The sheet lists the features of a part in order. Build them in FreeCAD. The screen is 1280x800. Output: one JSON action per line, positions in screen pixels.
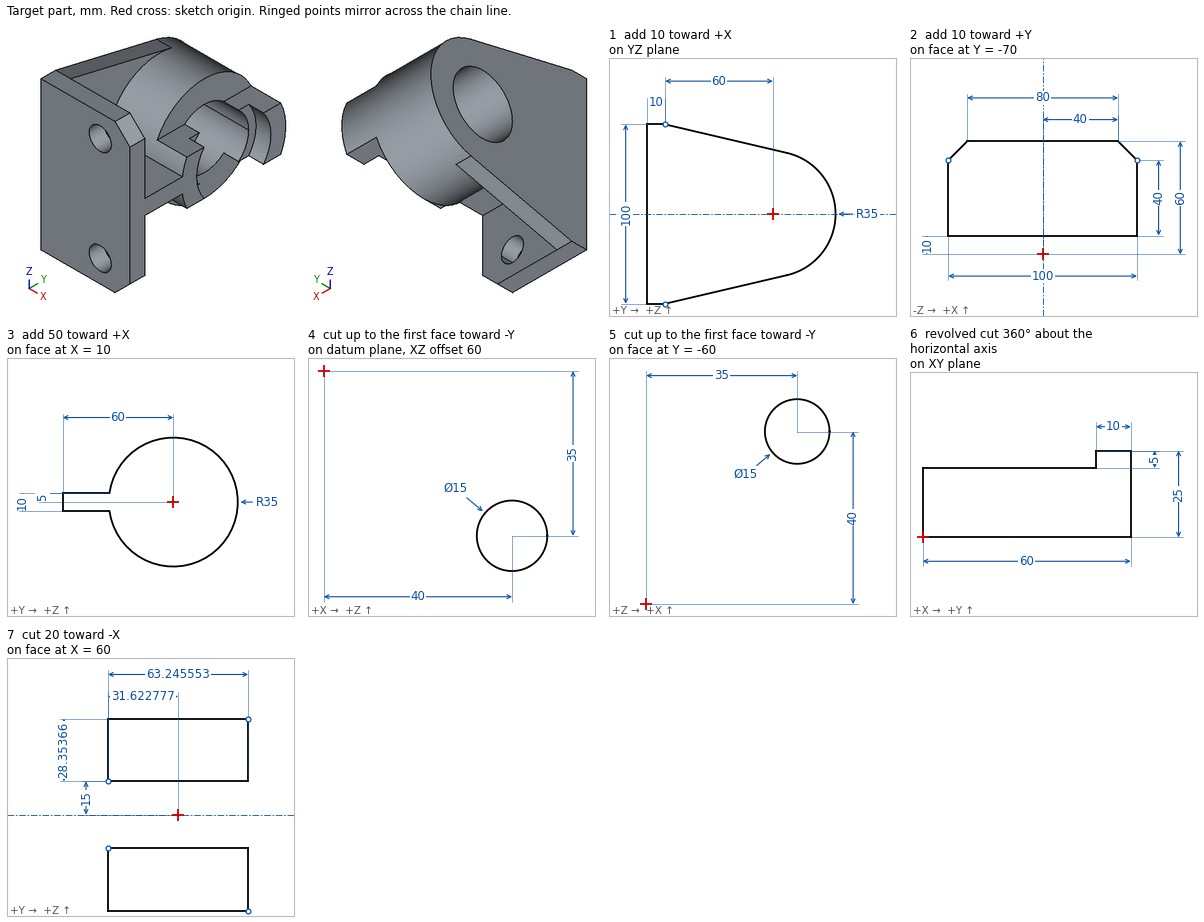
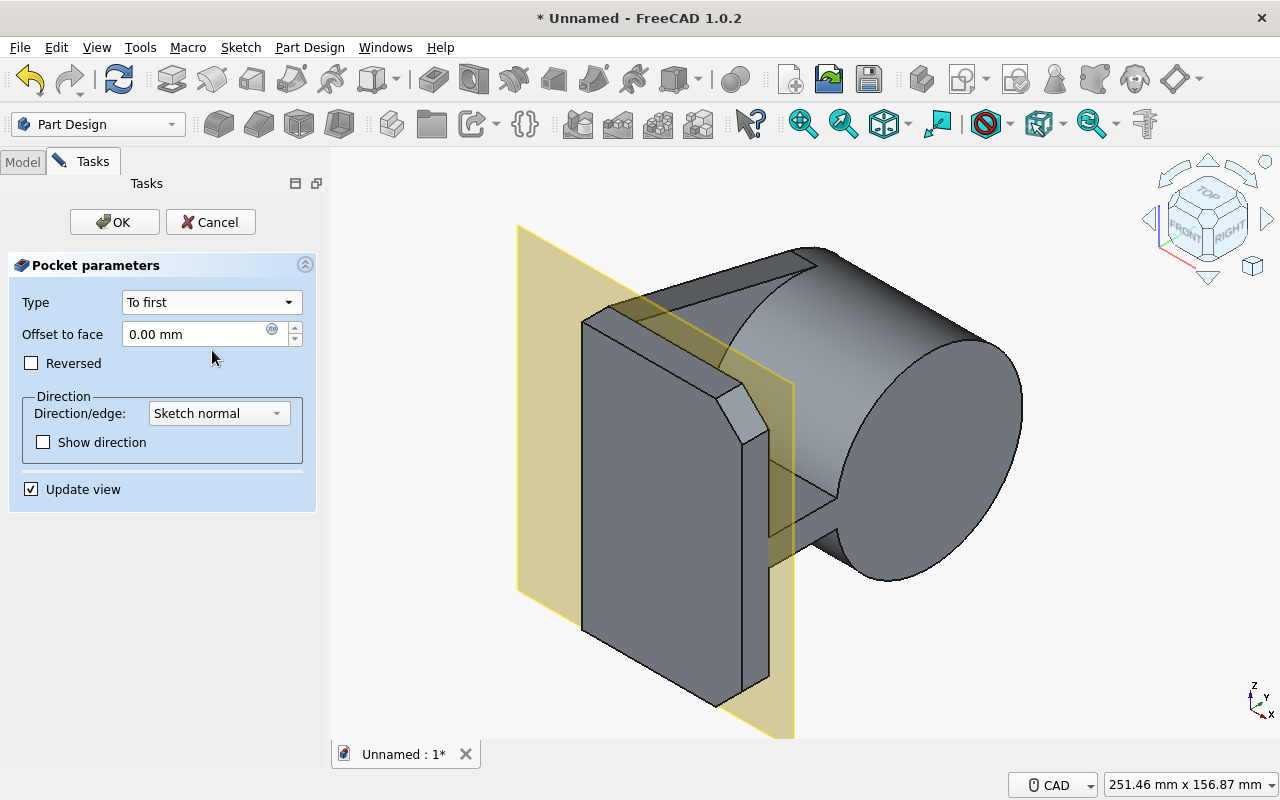
{"action": "left_click", "coordinate": [30, 363]}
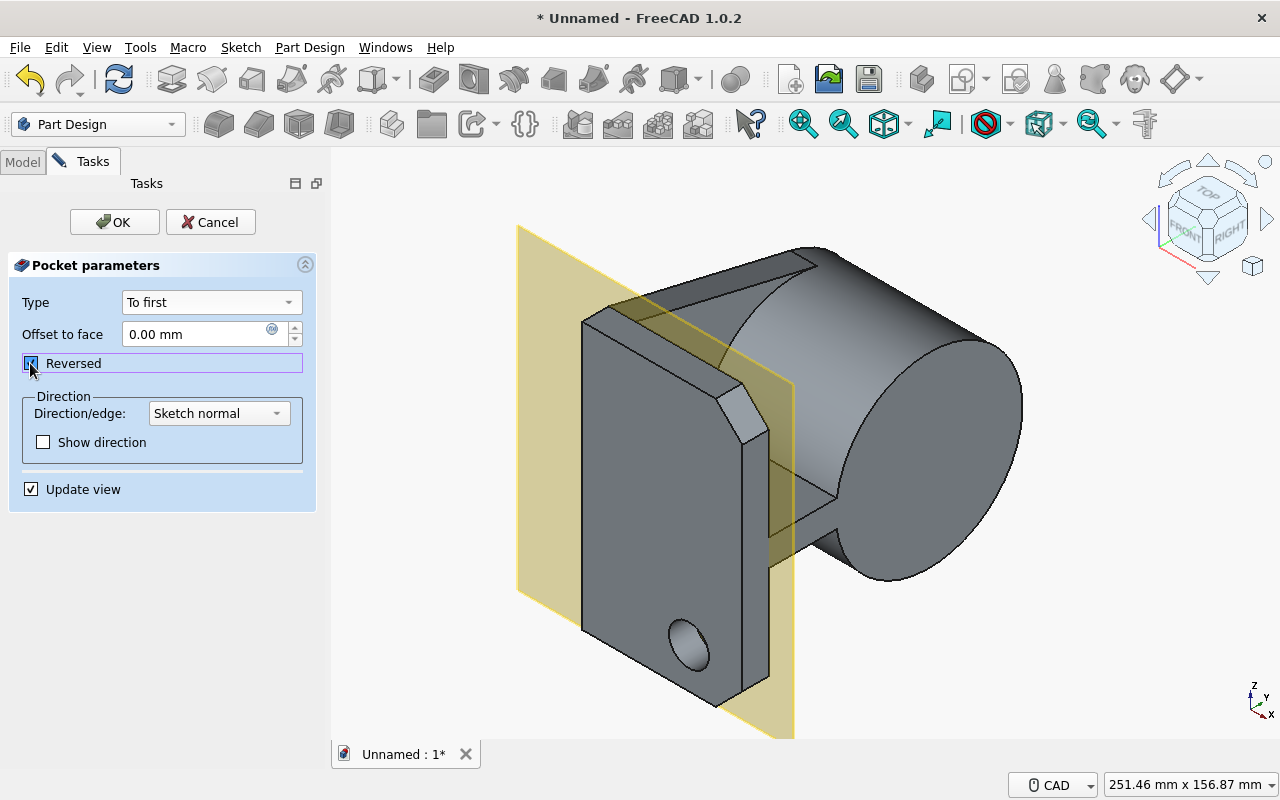
{"action": "left_click", "coordinate": [115, 222]}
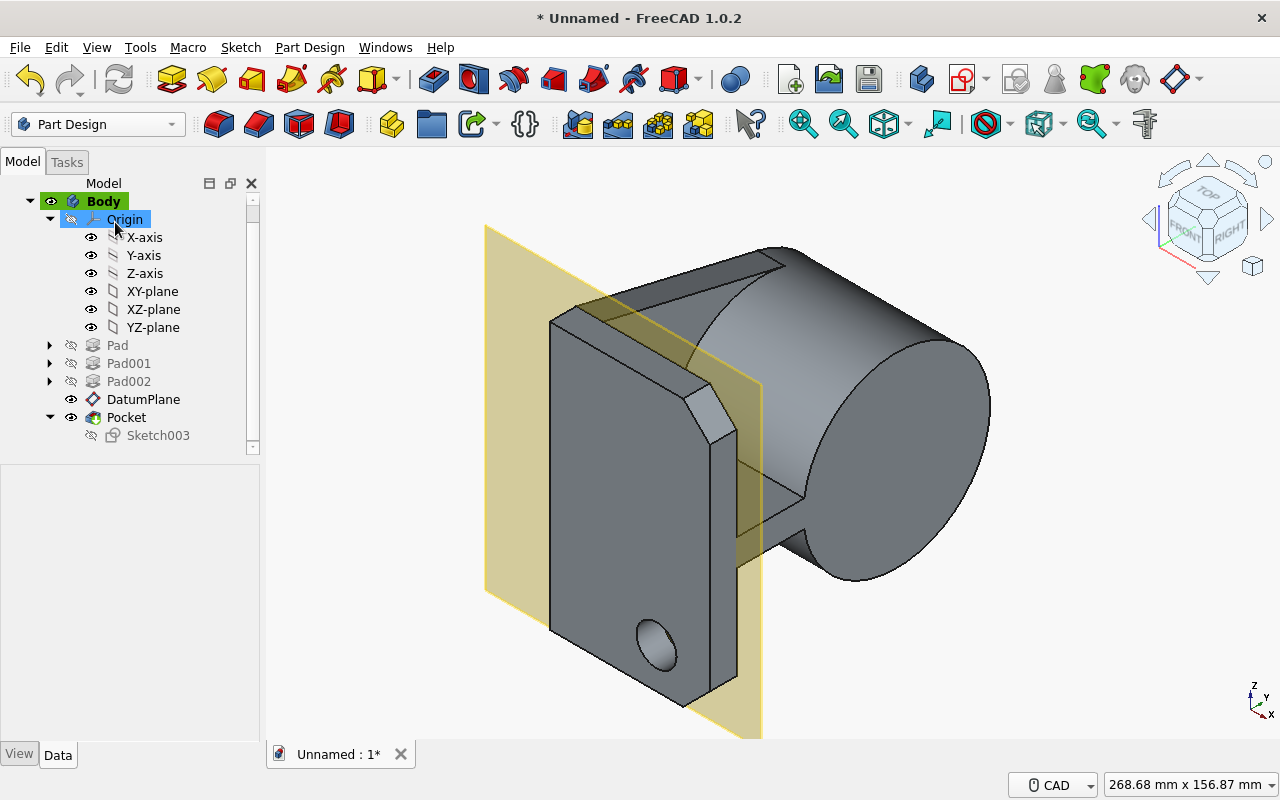
{"action": "left_click", "coordinate": [116, 399]}
{"action": "key", "text": "space"}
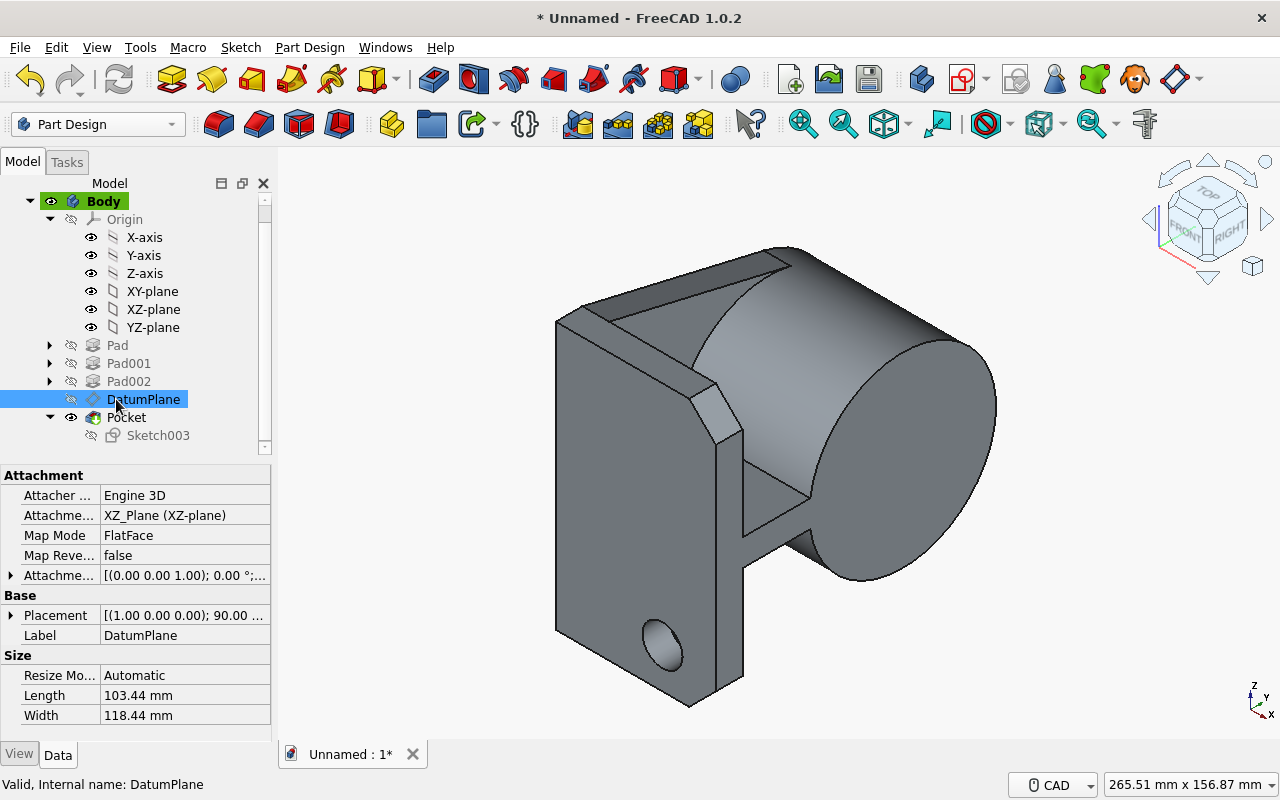
{"action": "key", "text": "4"}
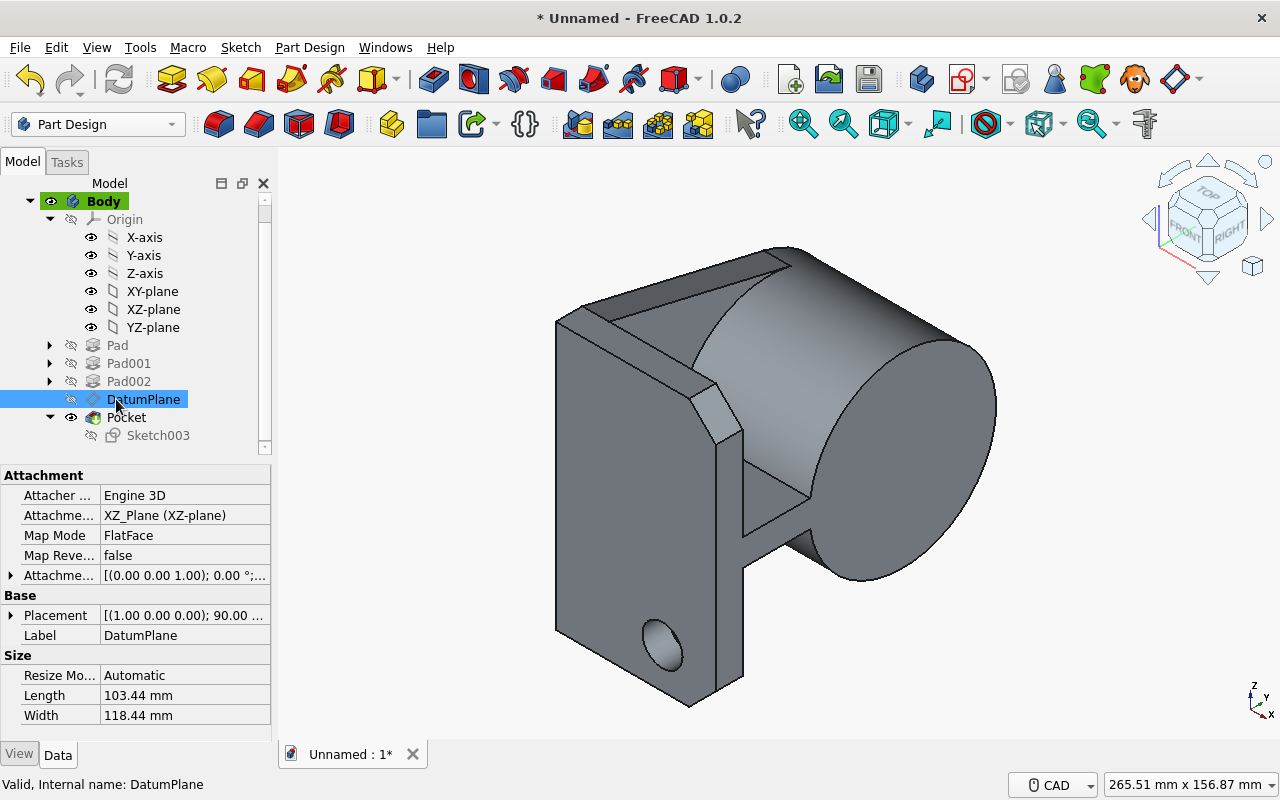
{"action": "left_click", "coordinate": [800, 576]}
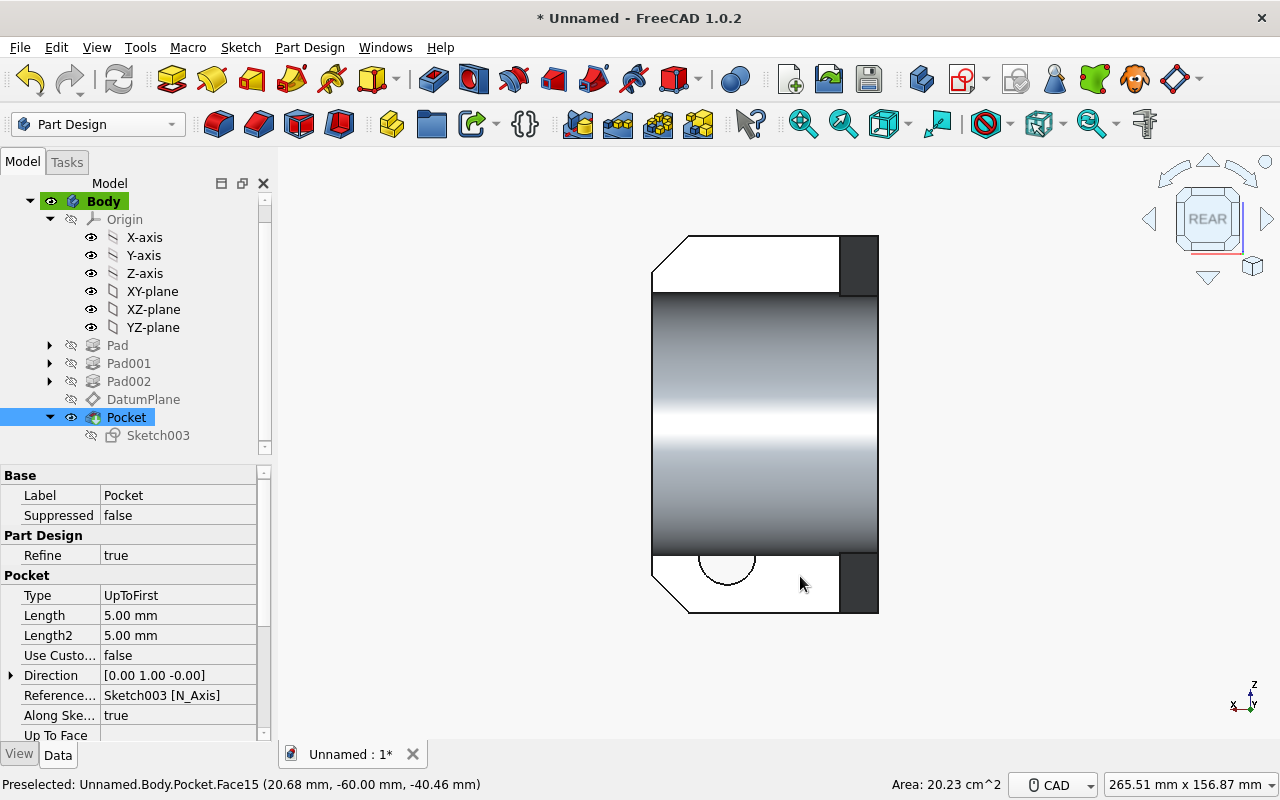
{"action": "left_click", "coordinate": [962, 80]}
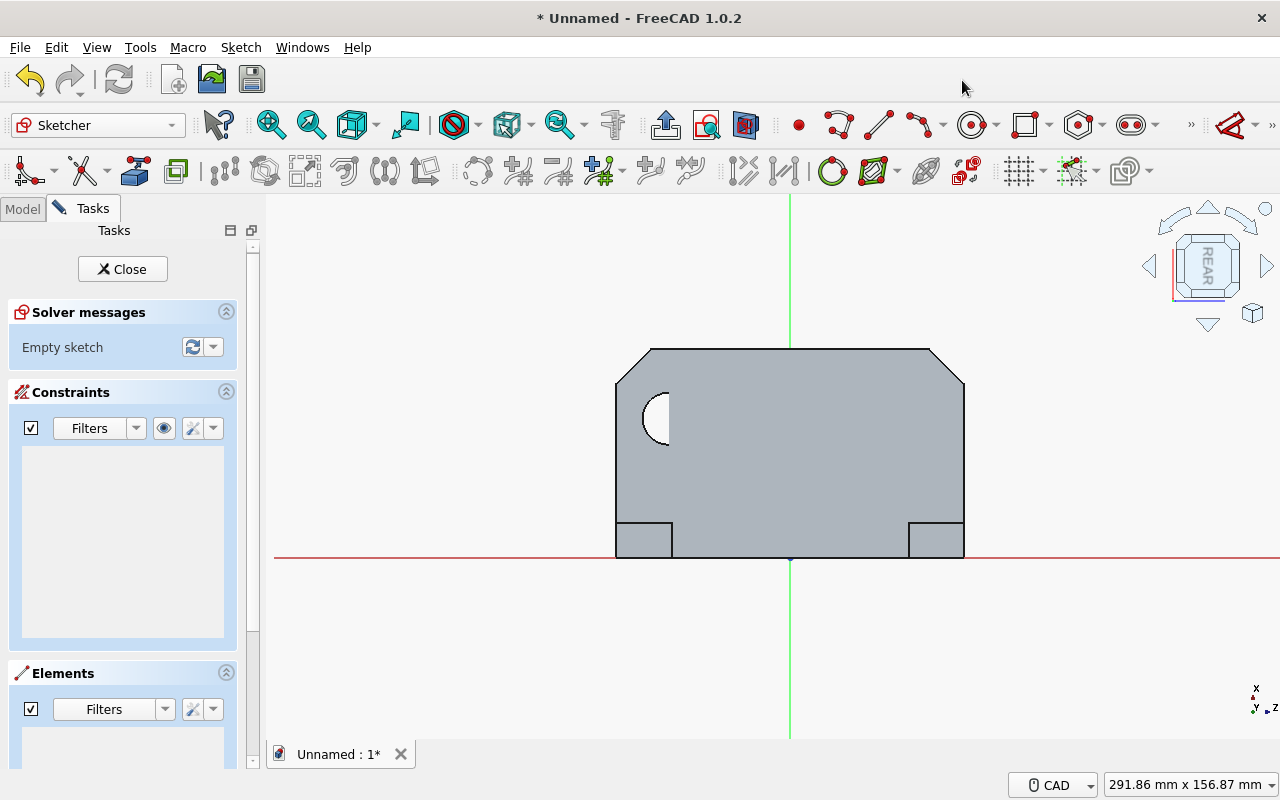
{"action": "left_click", "coordinate": [746, 126]}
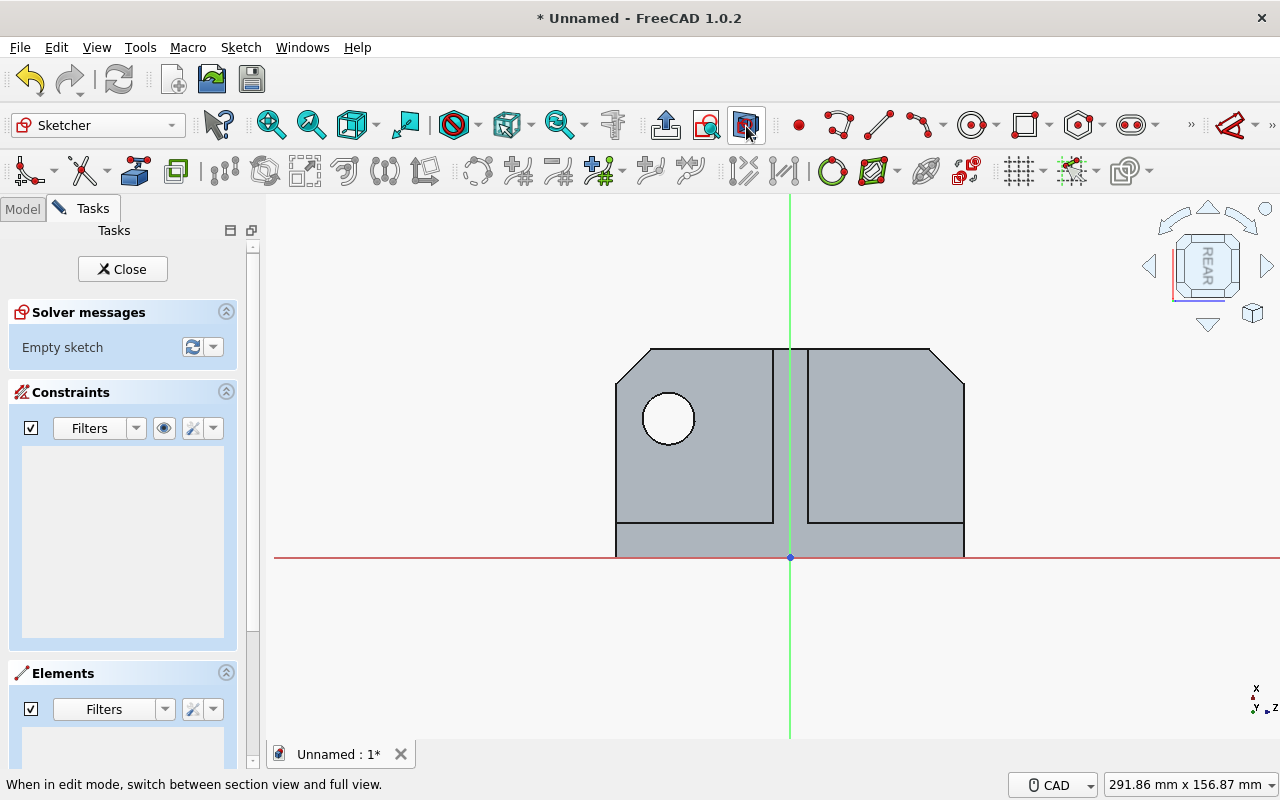
{"action": "scroll", "coordinate": [953, 409], "scroll_direction": "up", "scroll_amount": 9}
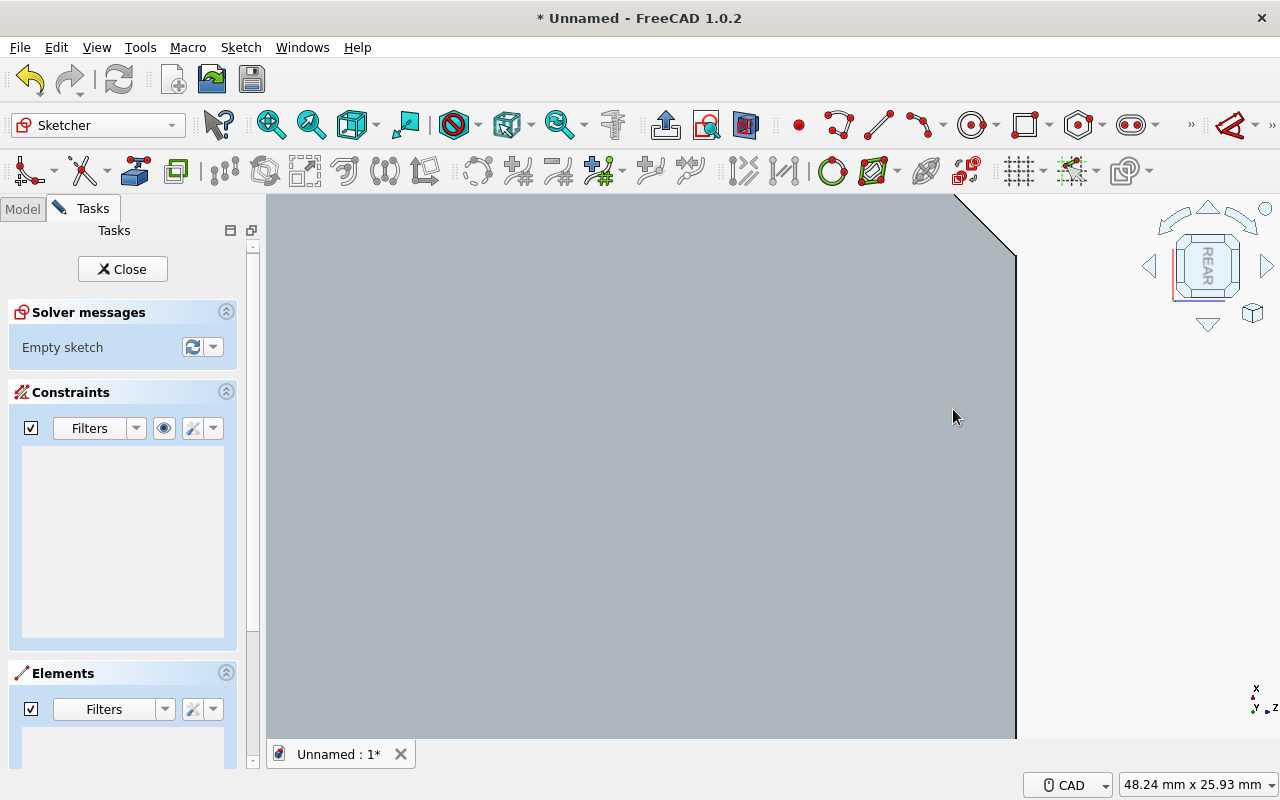
{"action": "key", "text": "g c"}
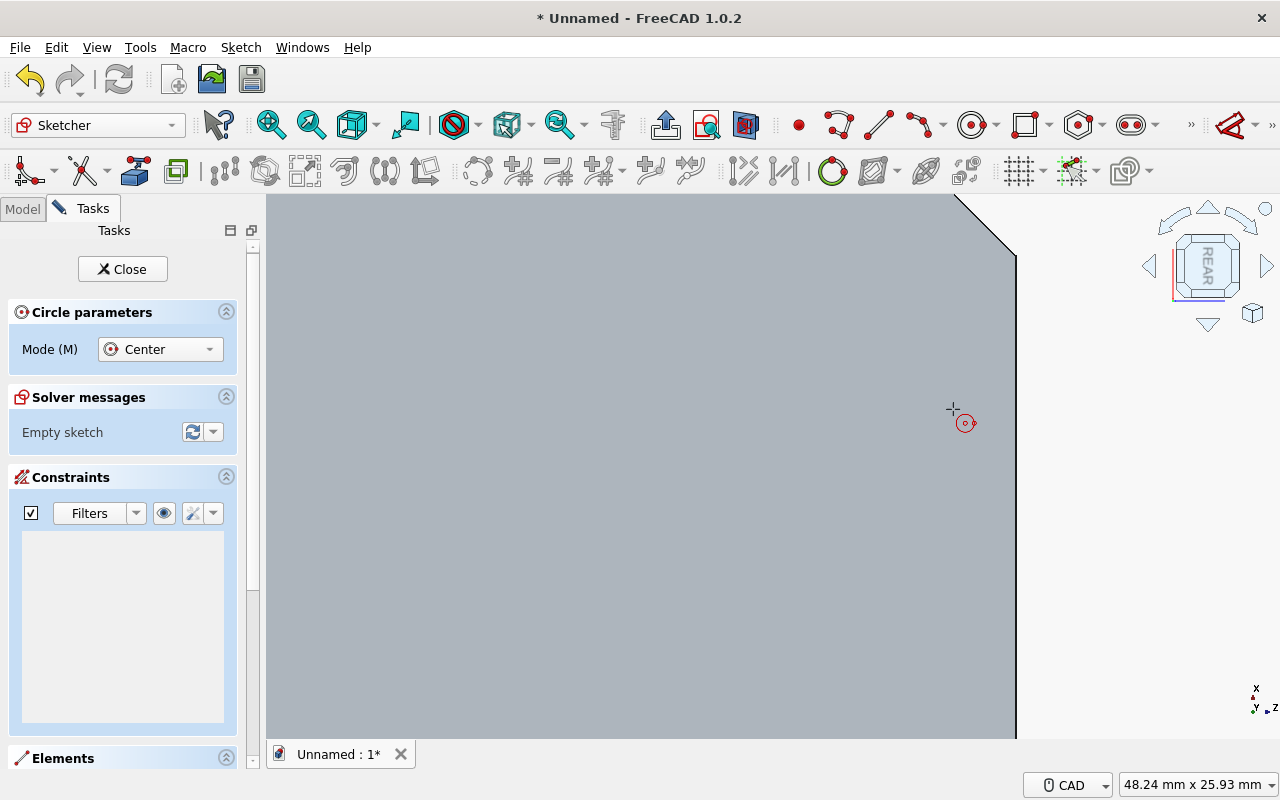
{"action": "left_click", "coordinate": [700, 466]}
{"action": "left_click", "coordinate": [812, 354]}
{"action": "key", "text": "Escape"}